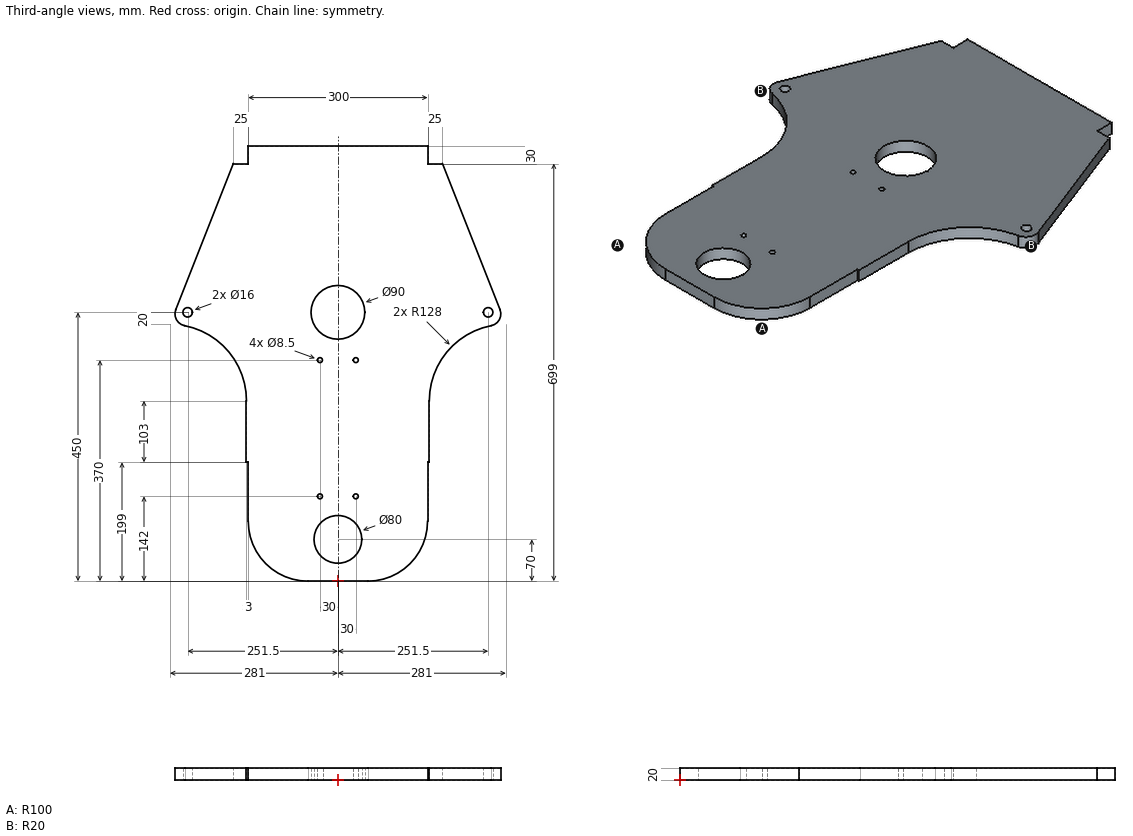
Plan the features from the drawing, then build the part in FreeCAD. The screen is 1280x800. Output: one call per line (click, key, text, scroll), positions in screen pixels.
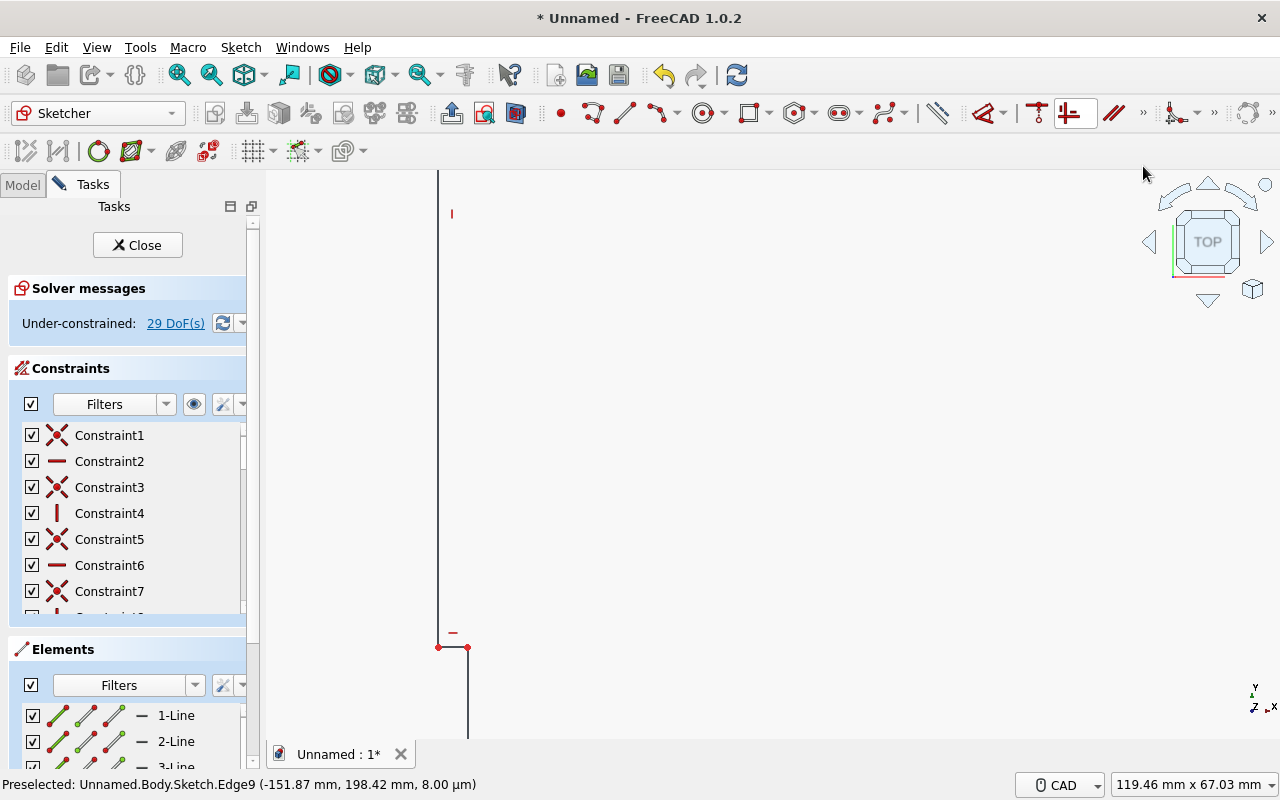
scroll(637, 534, down, 14)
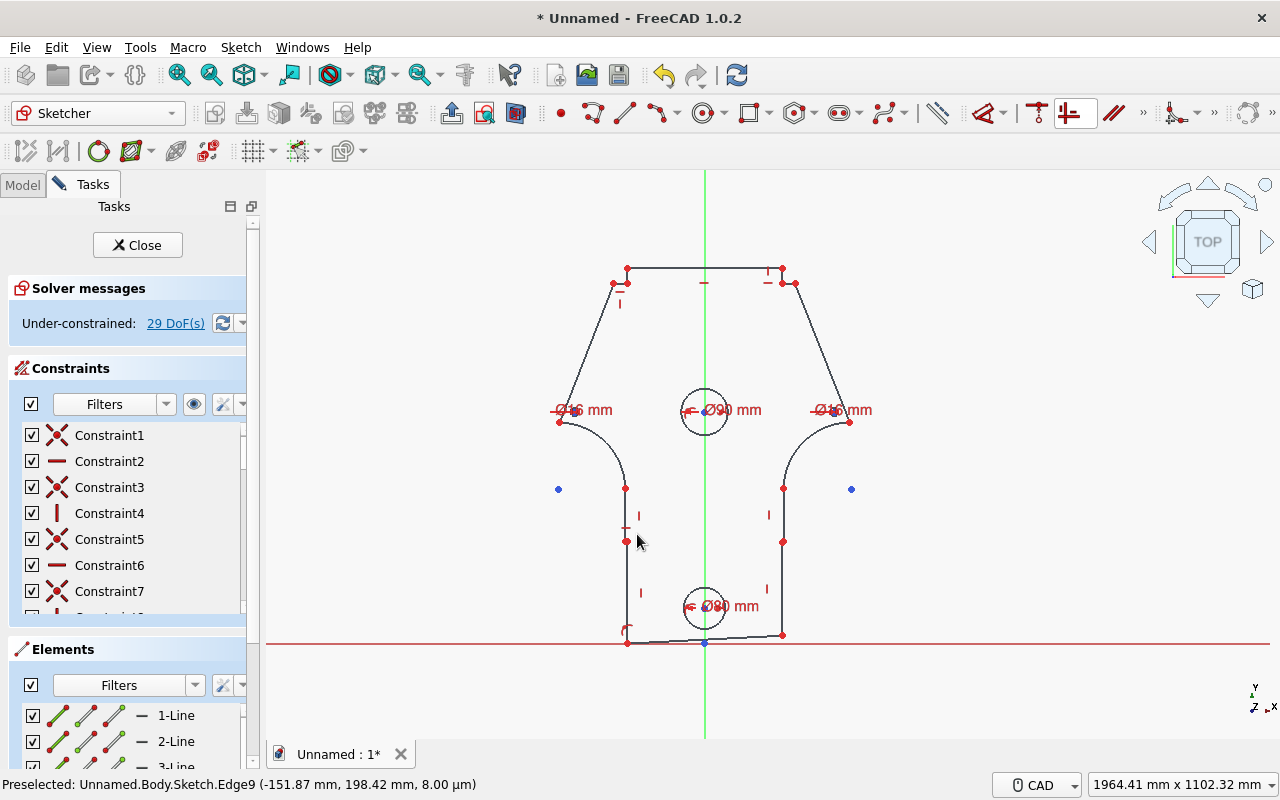
scroll(674, 641, up, 9)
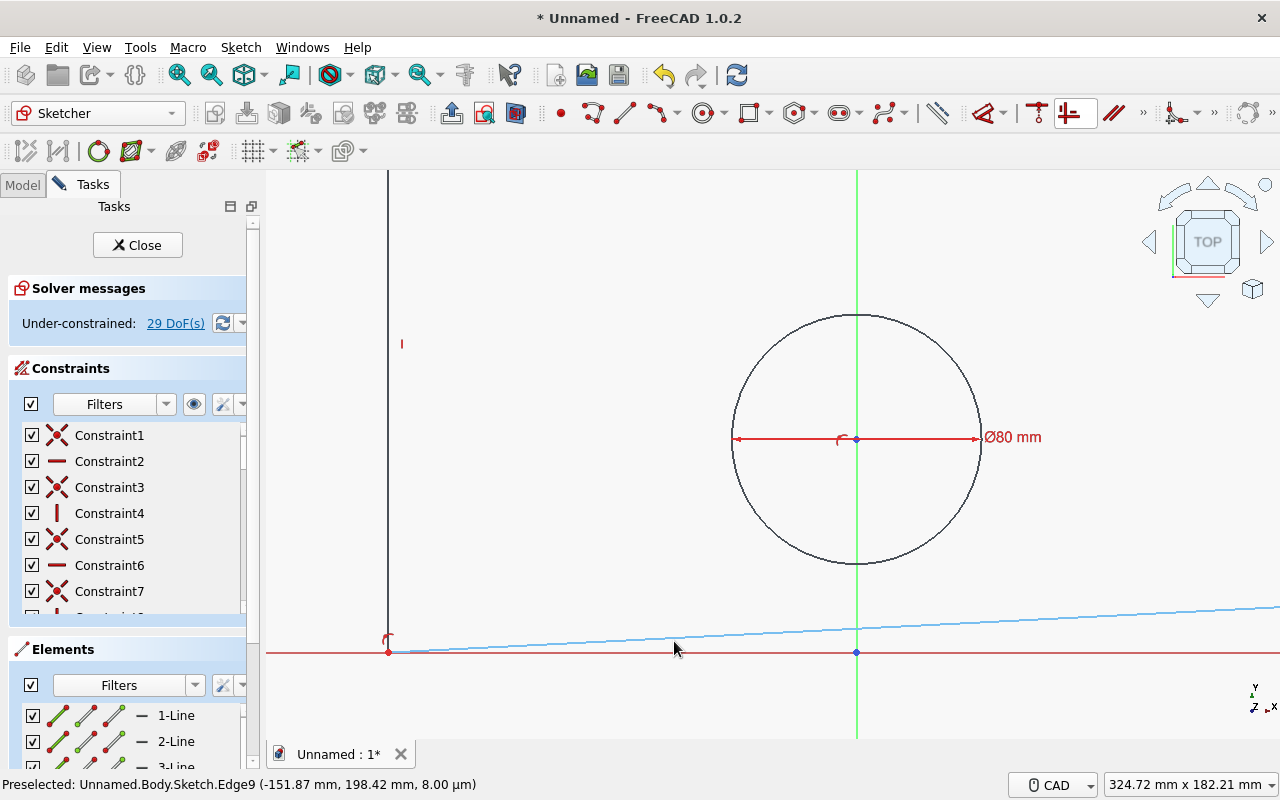
click(670, 638)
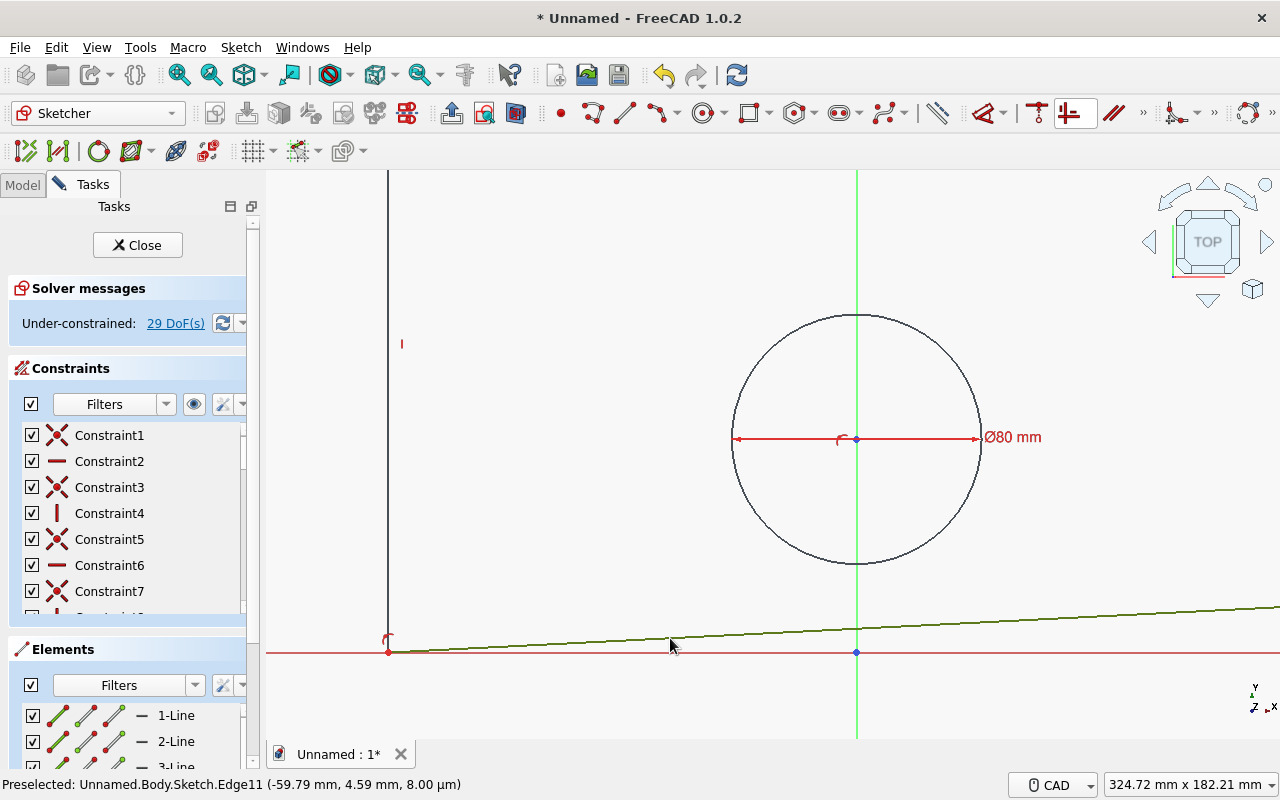
click(1092, 114)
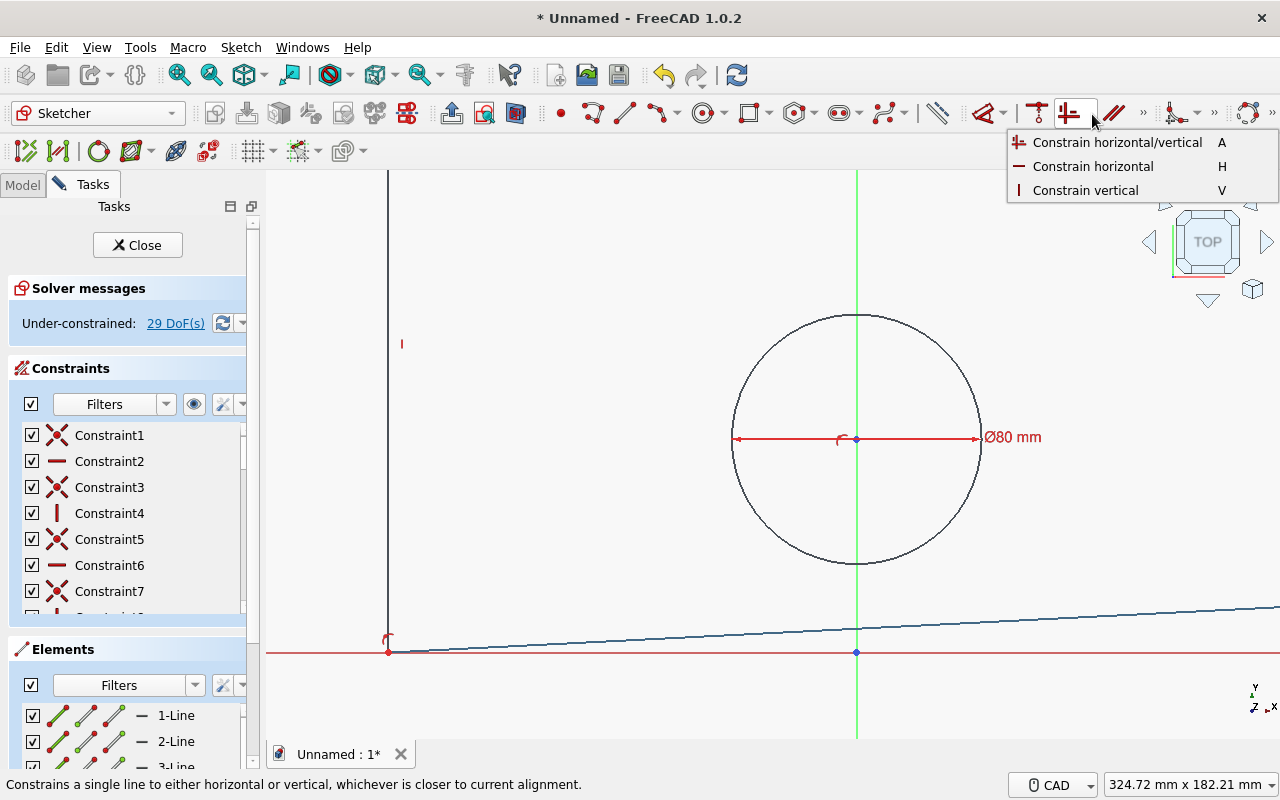
click(1143, 166)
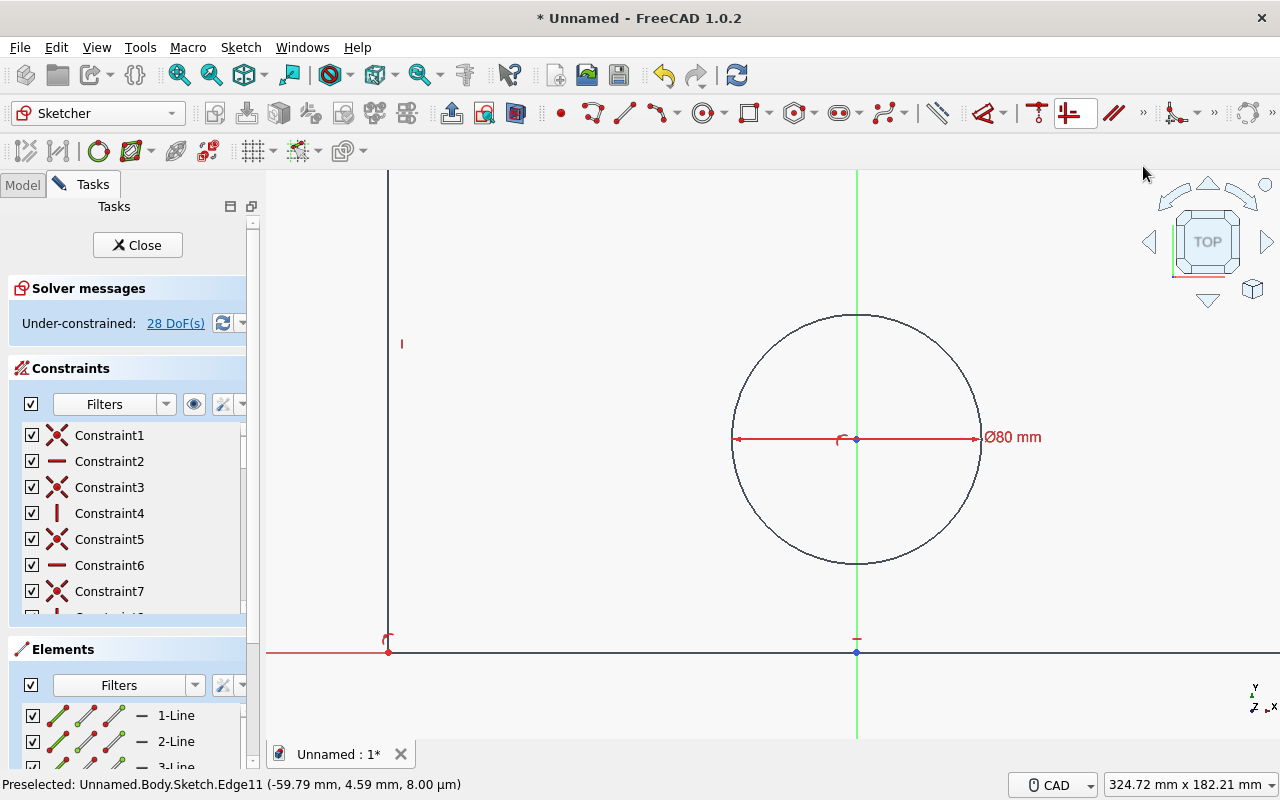
scroll(674, 641, down, 9)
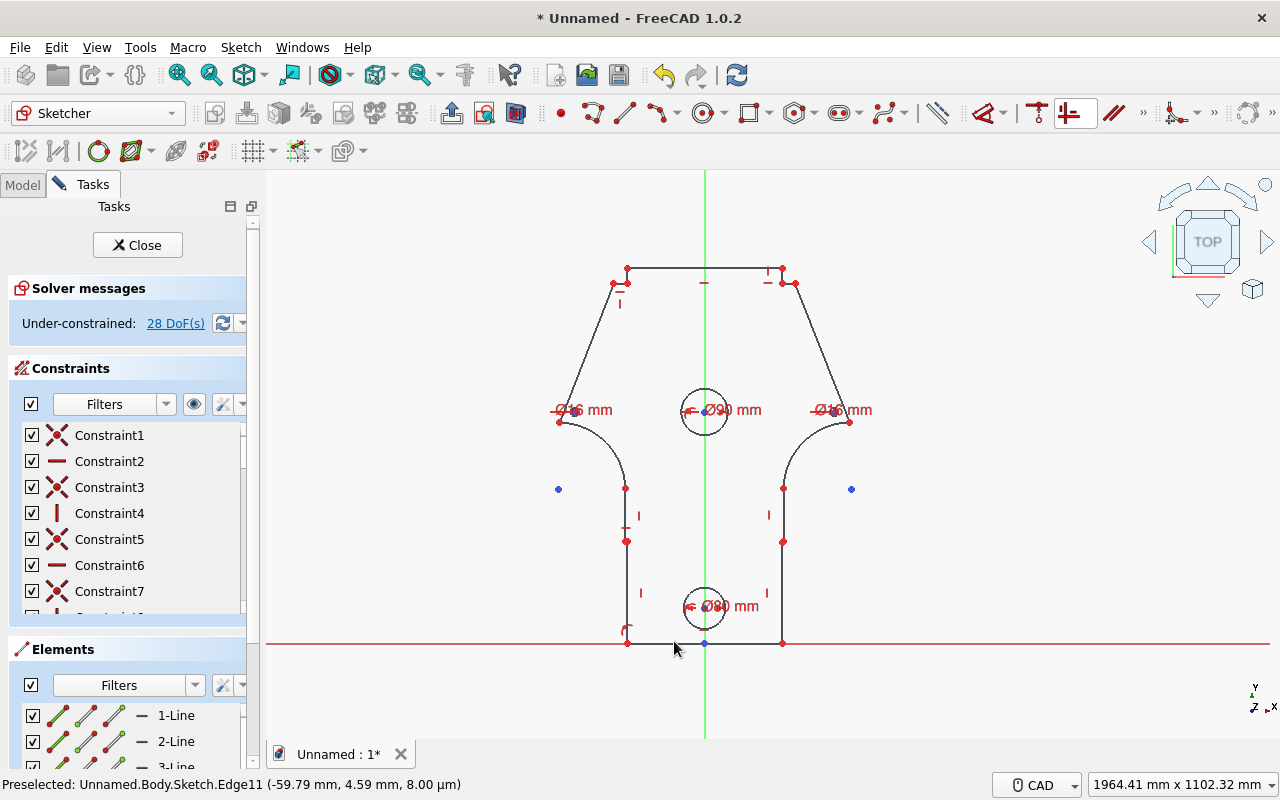
scroll(783, 542, up, 14)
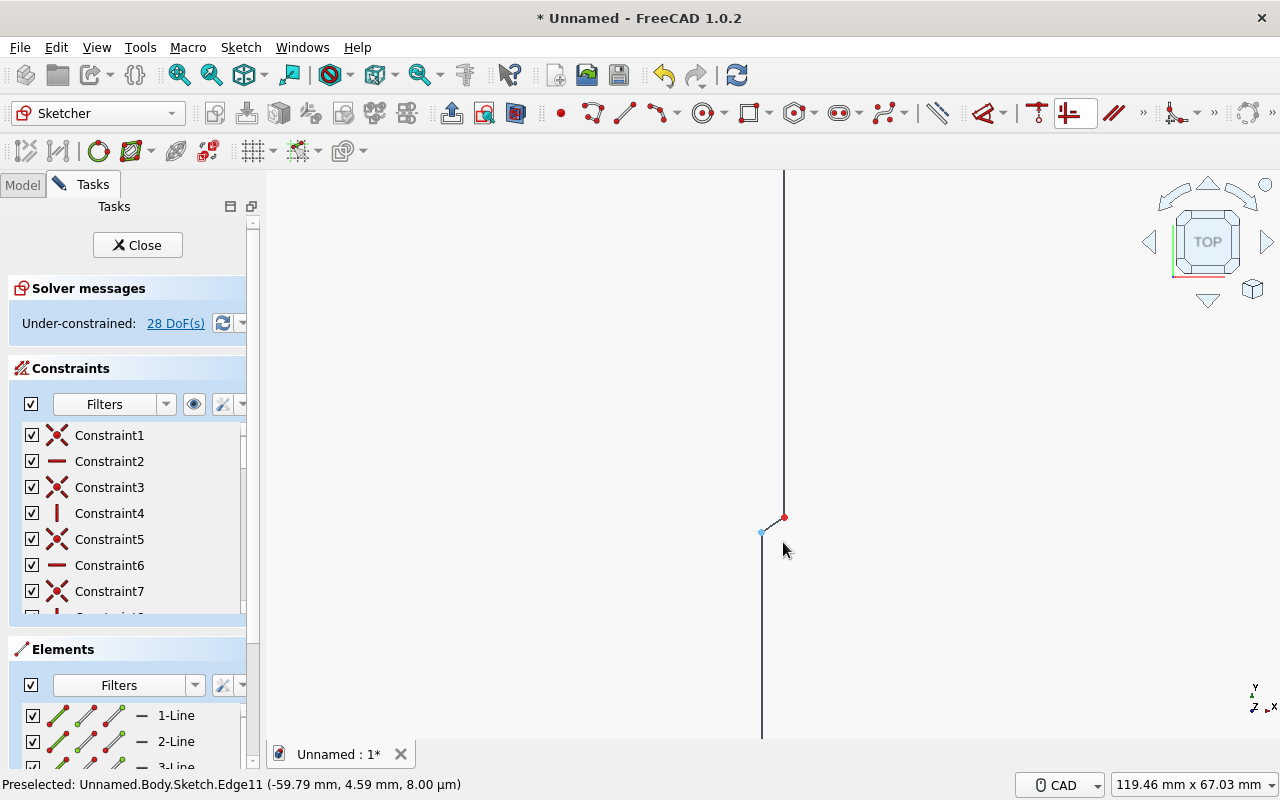
click(773, 525)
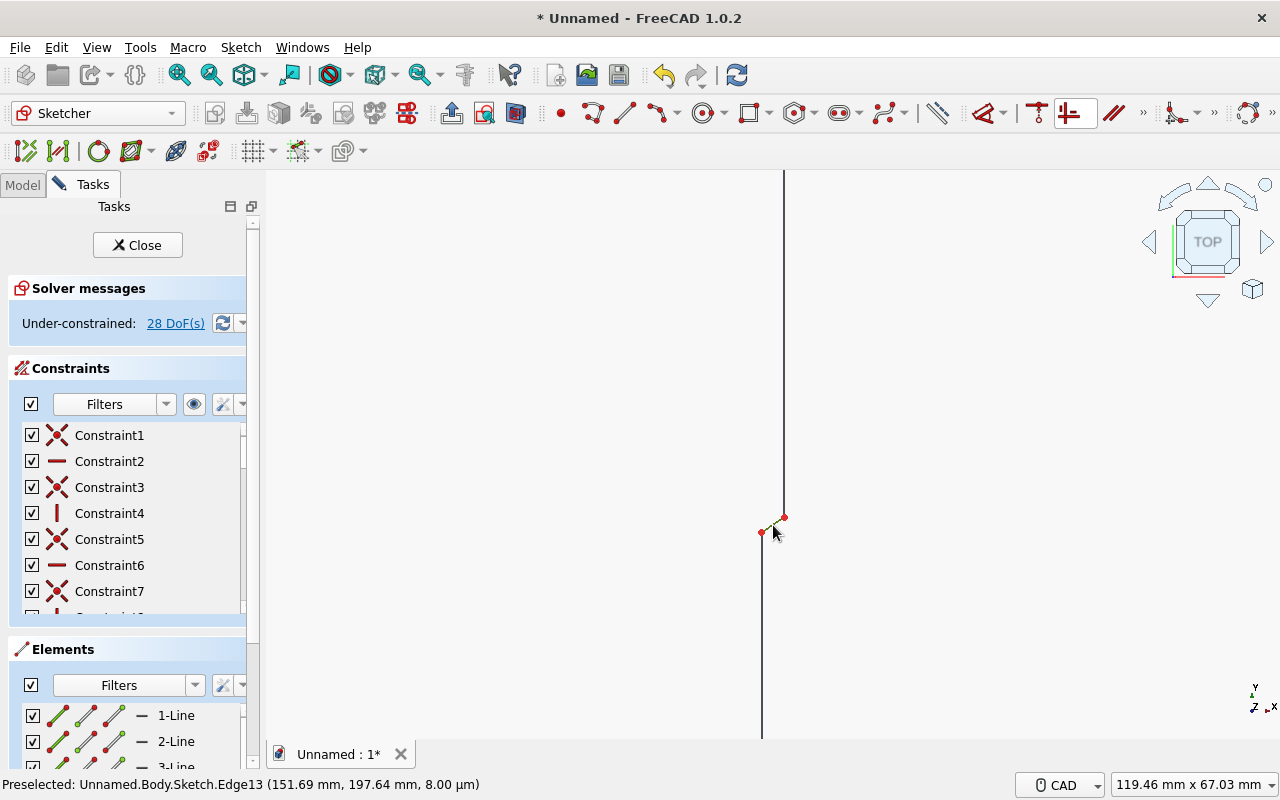
click(1092, 114)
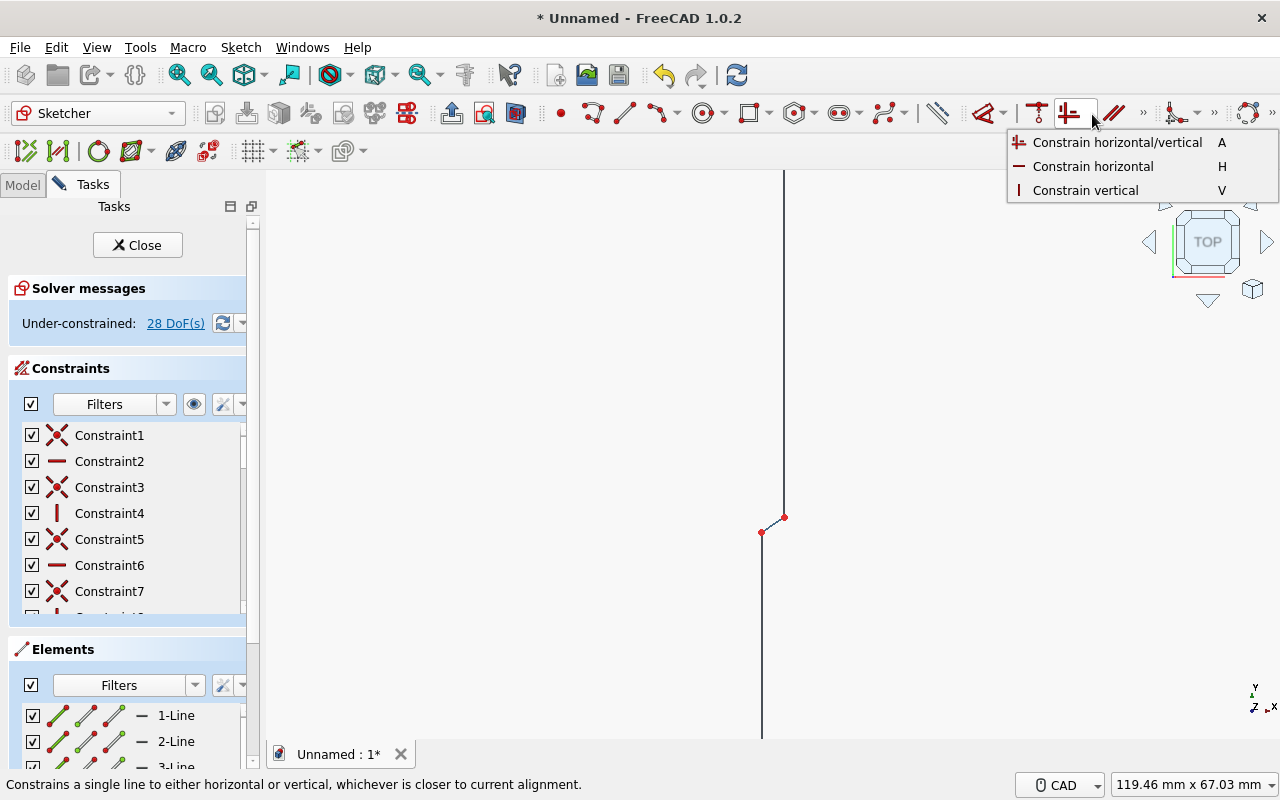
click(1143, 166)